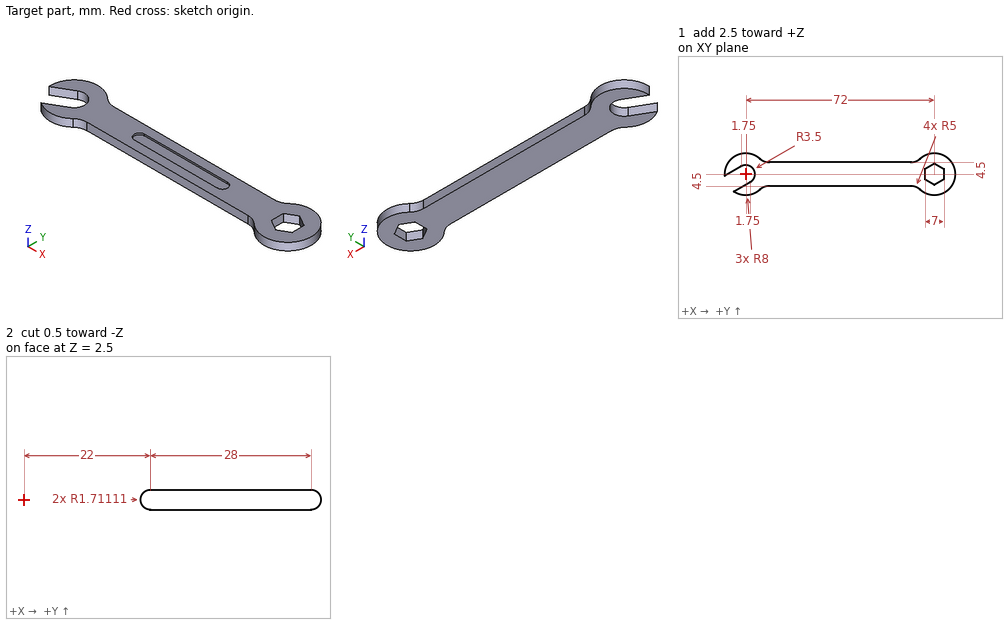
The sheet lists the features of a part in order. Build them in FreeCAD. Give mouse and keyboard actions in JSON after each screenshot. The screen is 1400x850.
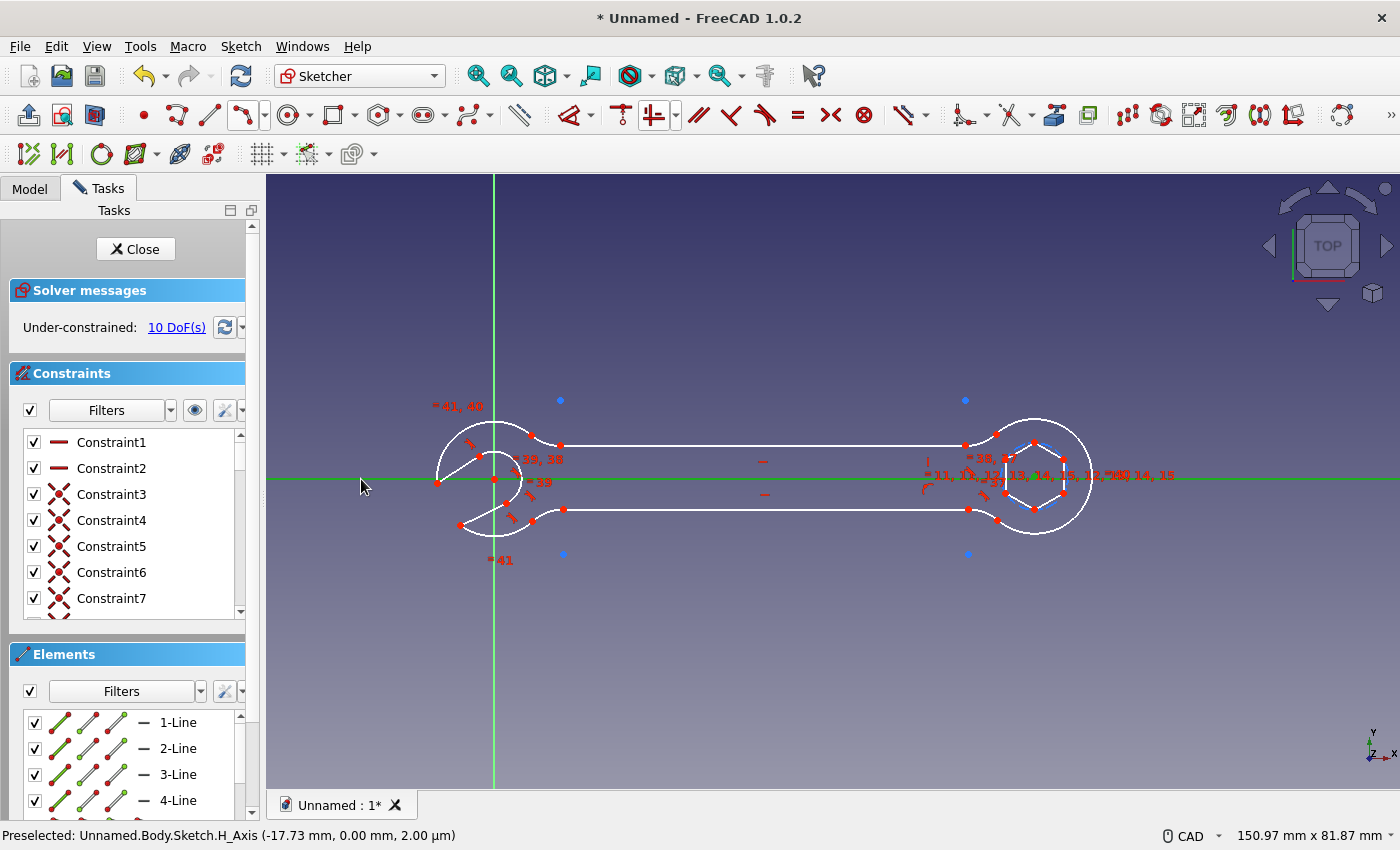
{"action": "key", "text": "c"}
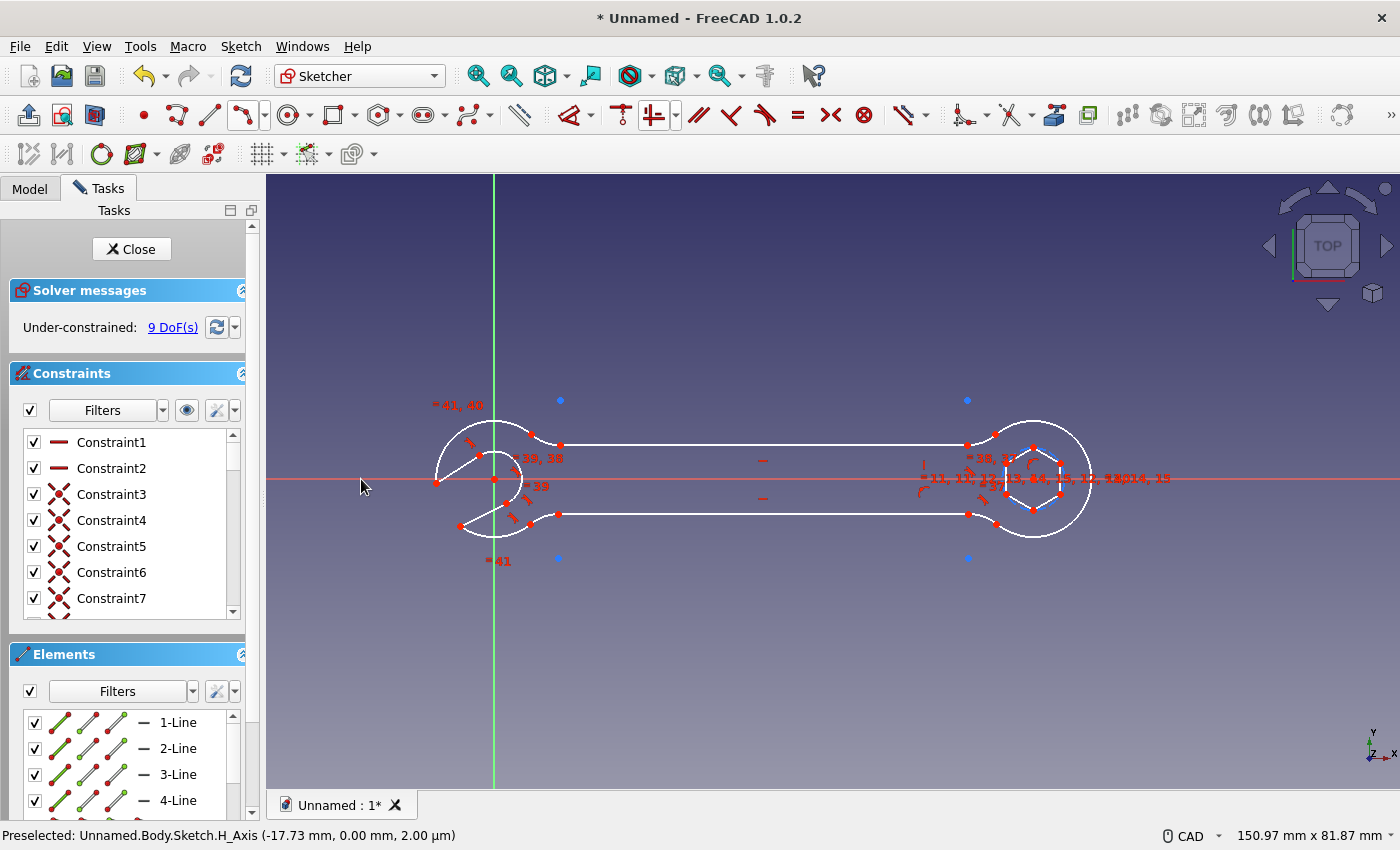
{"action": "scroll", "coordinate": [989, 519], "scroll_direction": "up", "scroll_amount": 3}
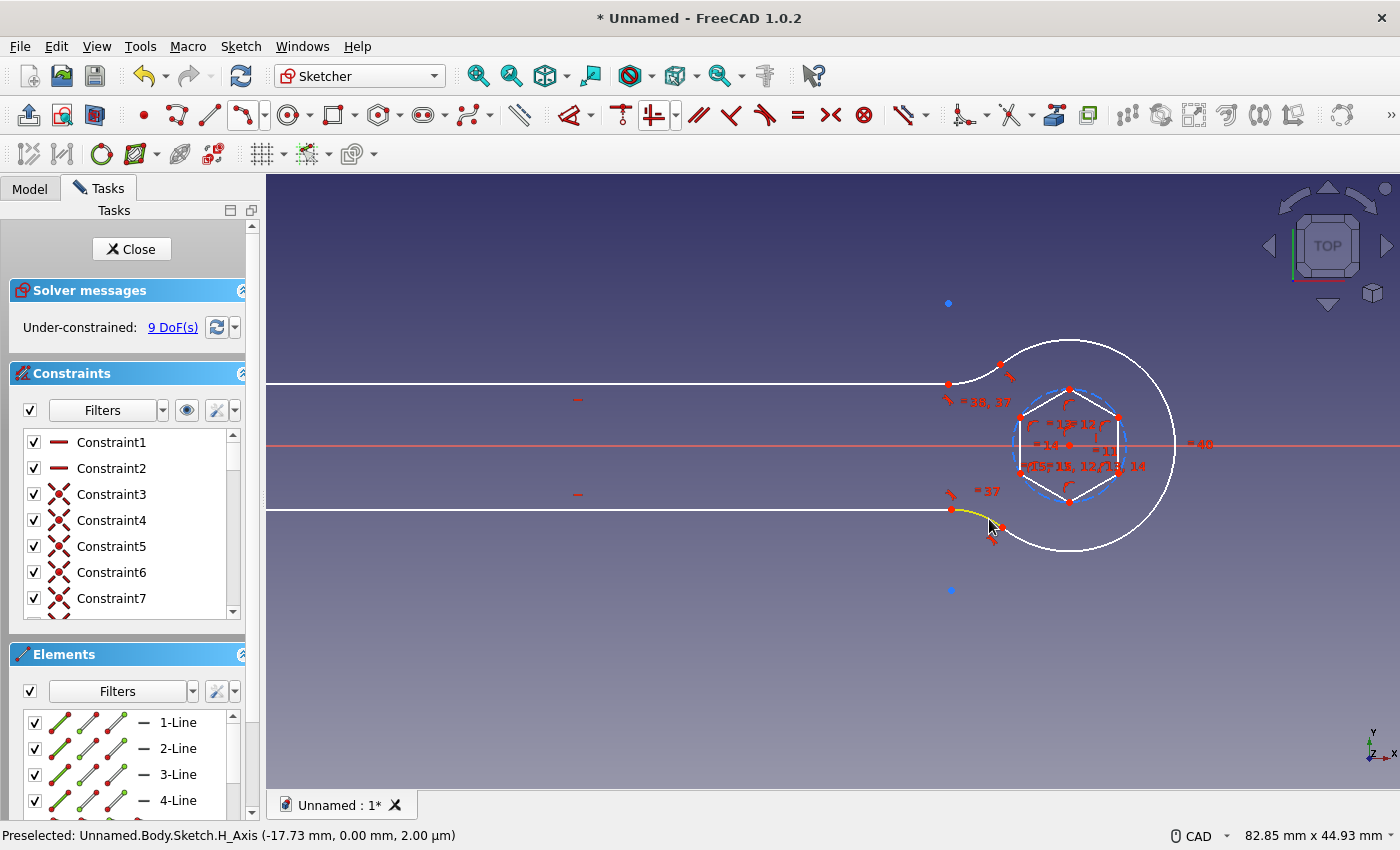
{"action": "left_click", "coordinate": [989, 519]}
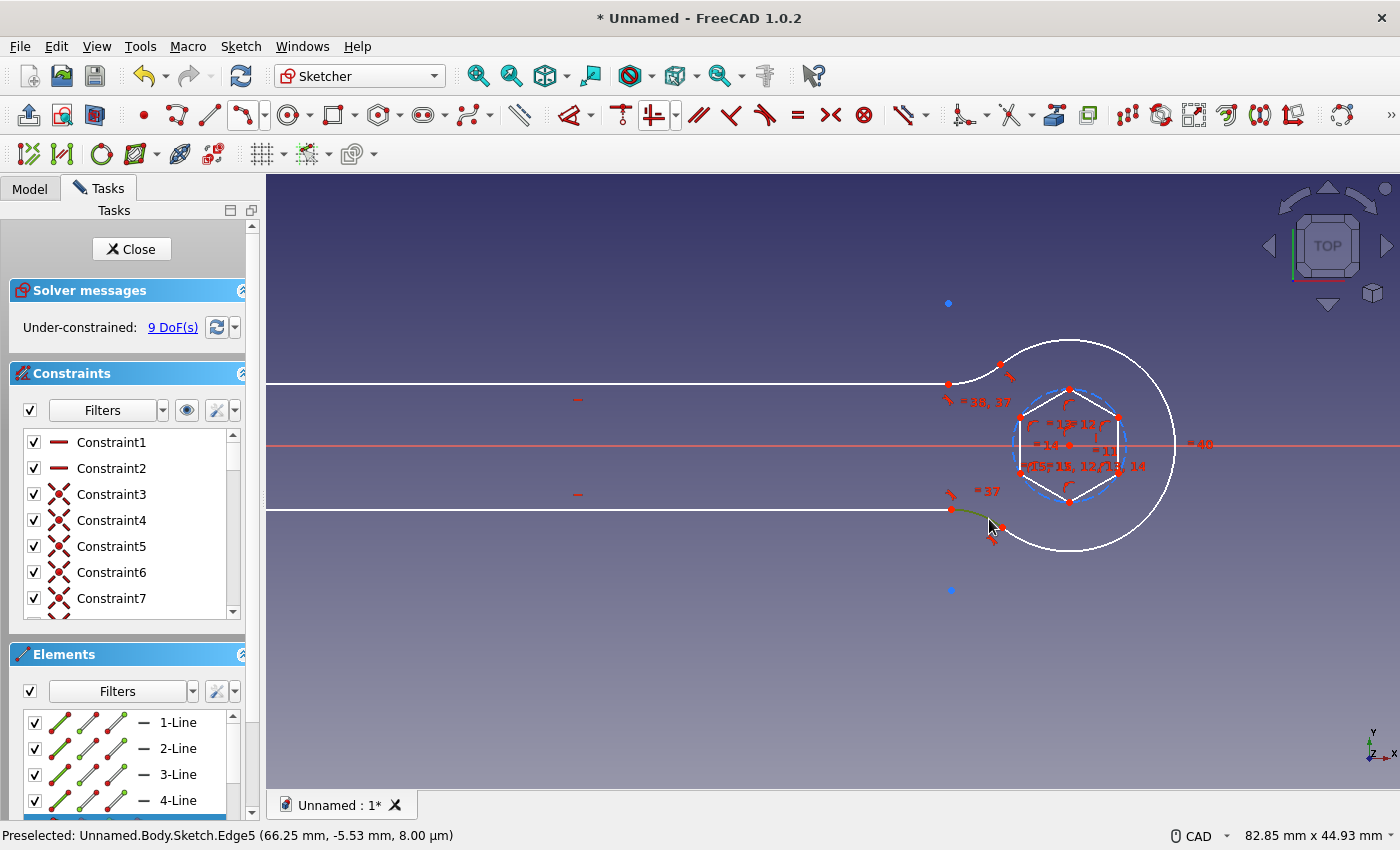
{"action": "left_click", "coordinate": [590, 116]}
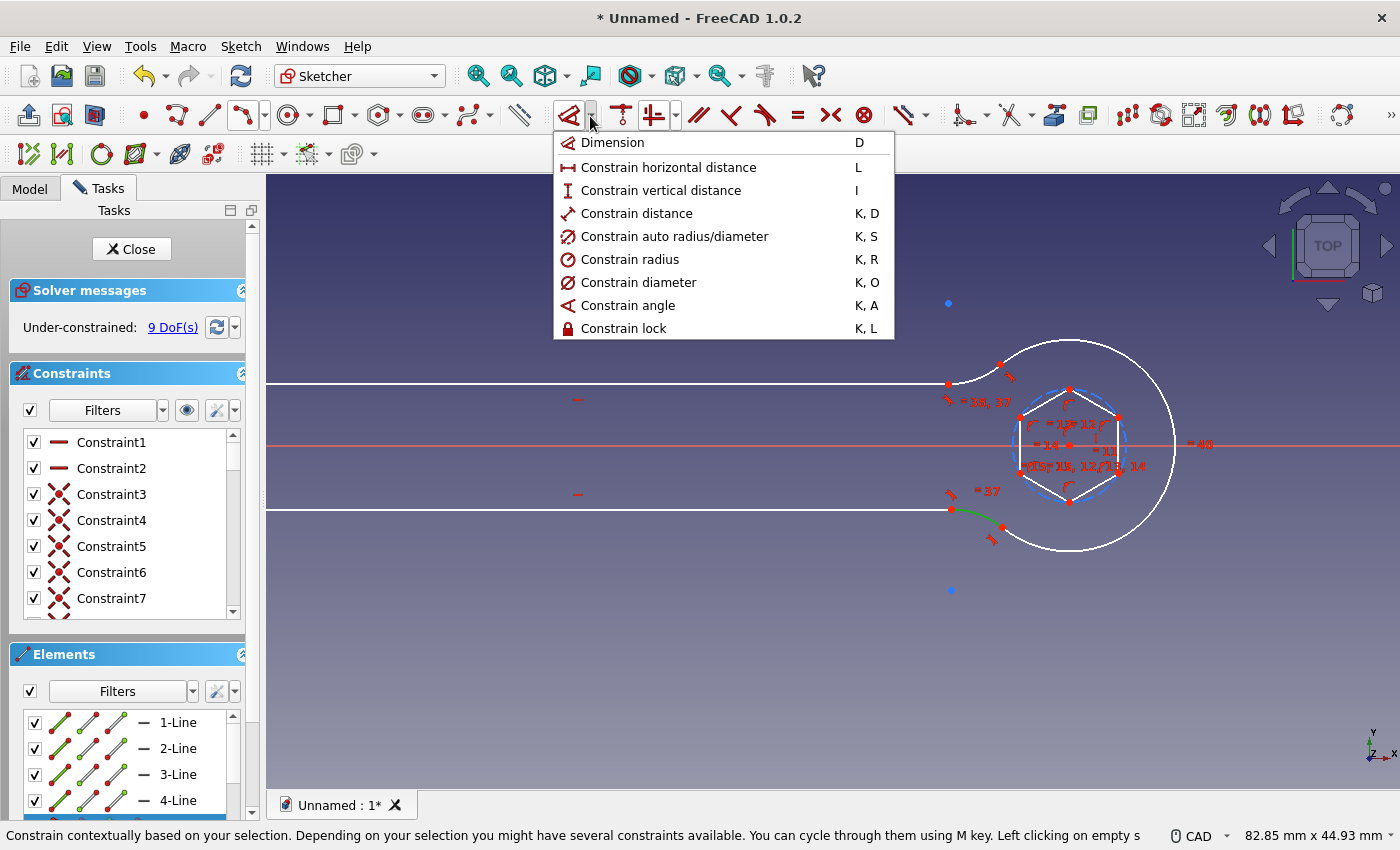
{"action": "left_click", "coordinate": [724, 260]}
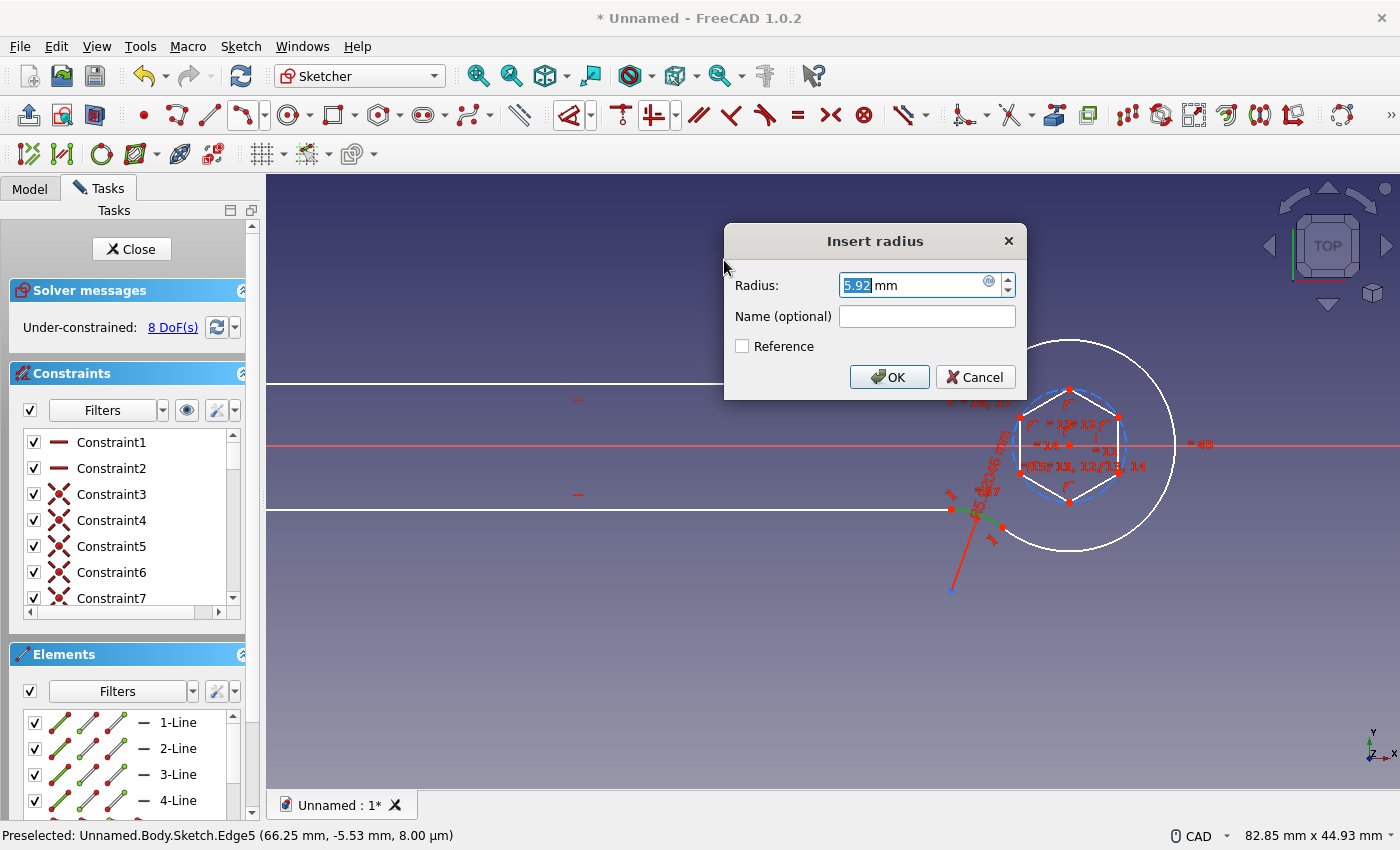
{"action": "type", "text": "5"}
{"action": "key", "text": "Return"}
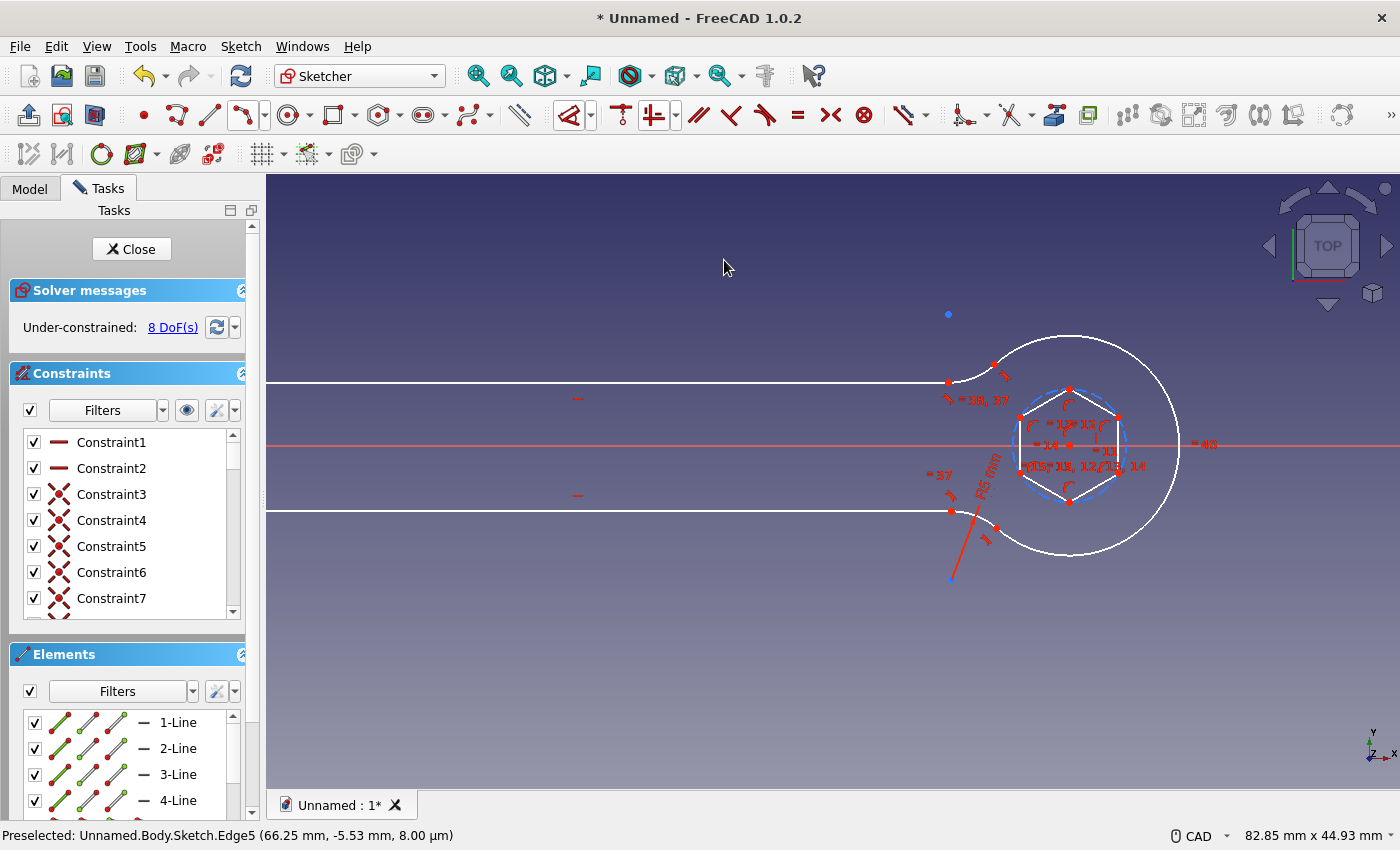
{"action": "left_click", "coordinate": [1137, 532]}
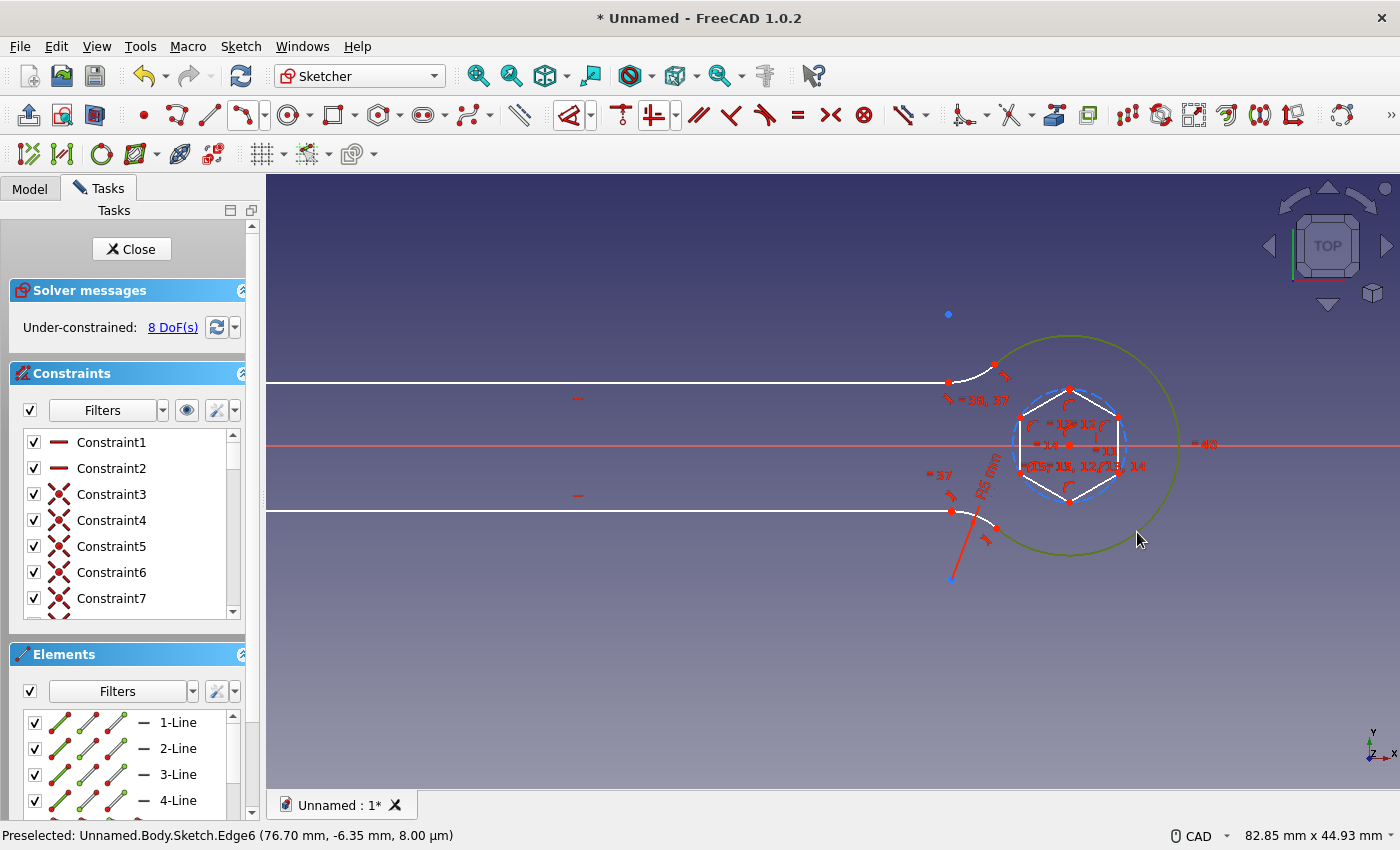
{"action": "key", "text": "k r"}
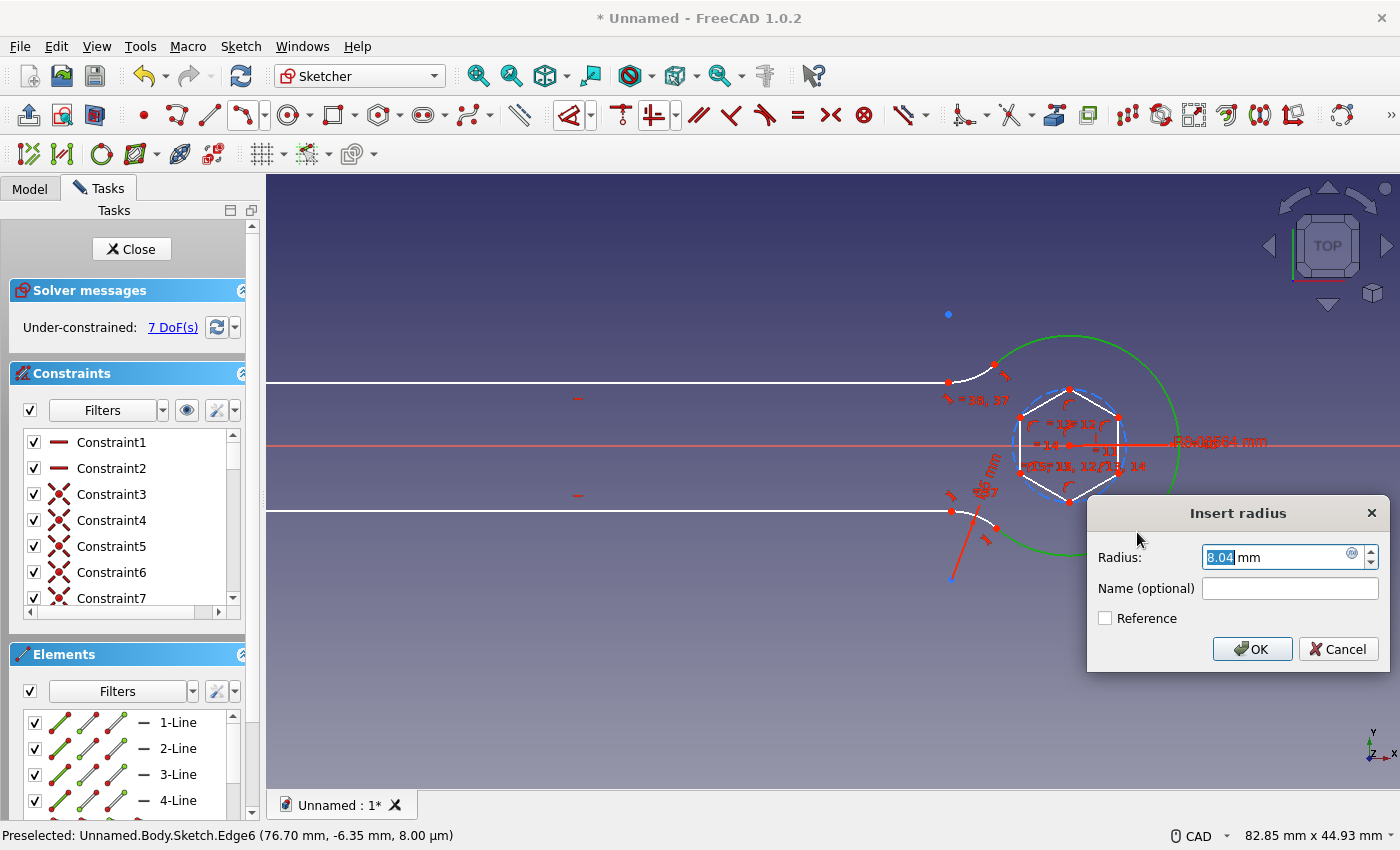
{"action": "type", "text": "8"}
{"action": "key", "text": "Return"}